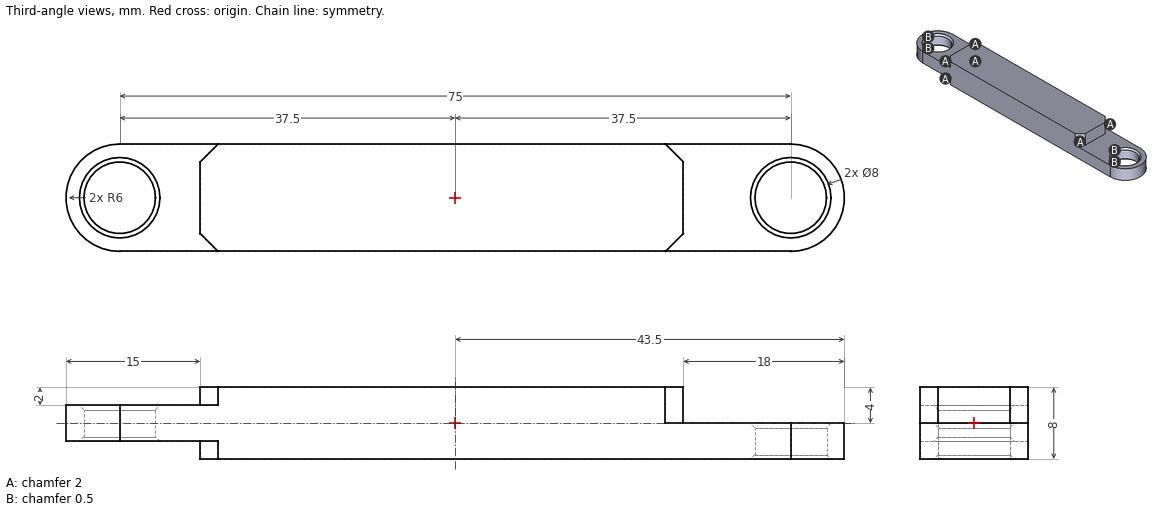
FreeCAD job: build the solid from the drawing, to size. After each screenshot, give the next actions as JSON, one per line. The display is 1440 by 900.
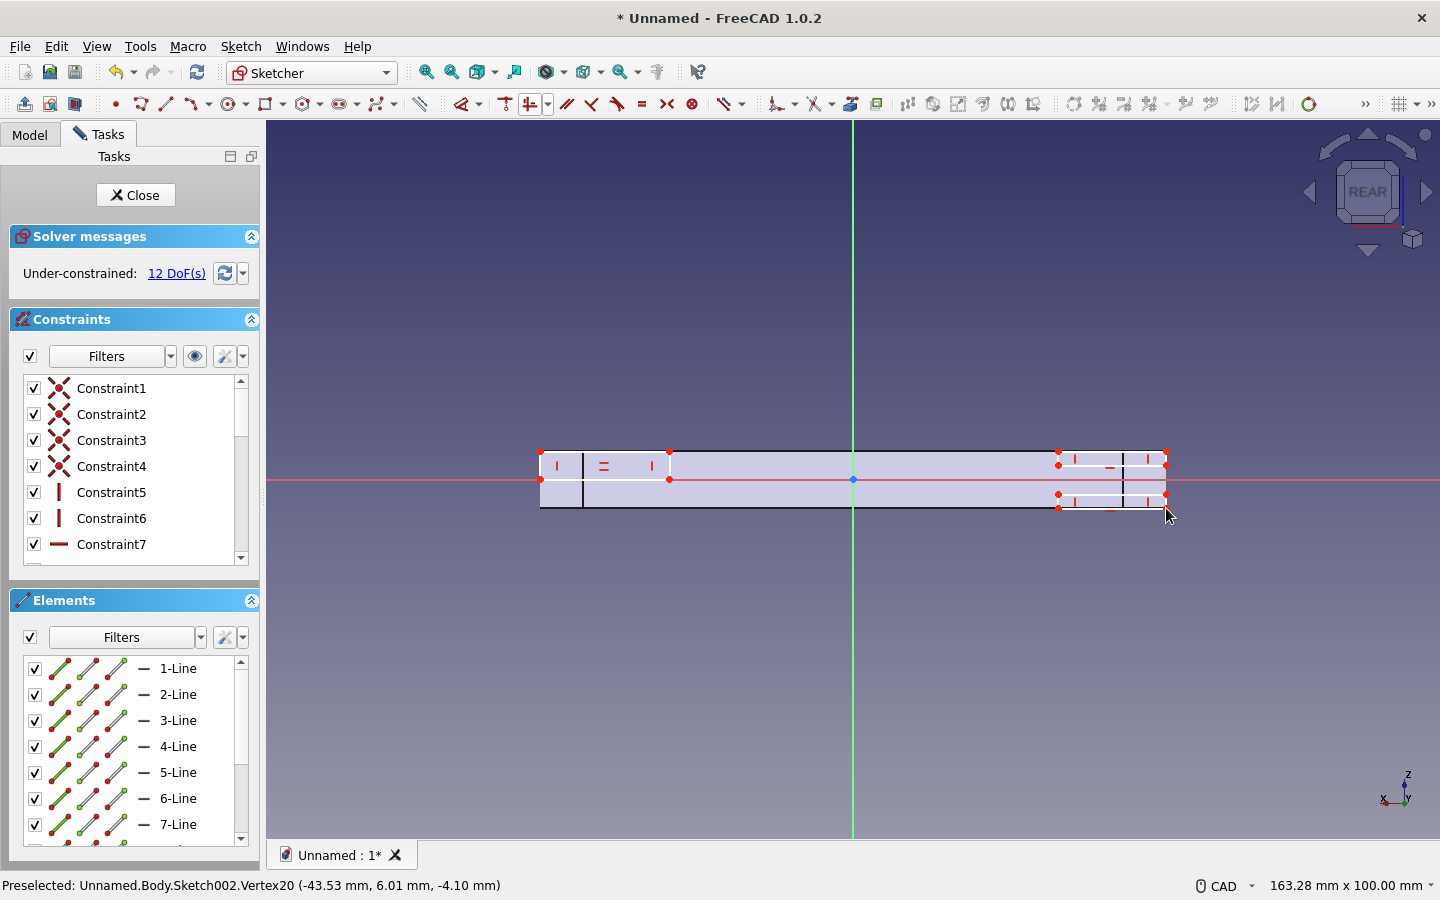
{"action": "left_click", "coordinate": [540, 452]}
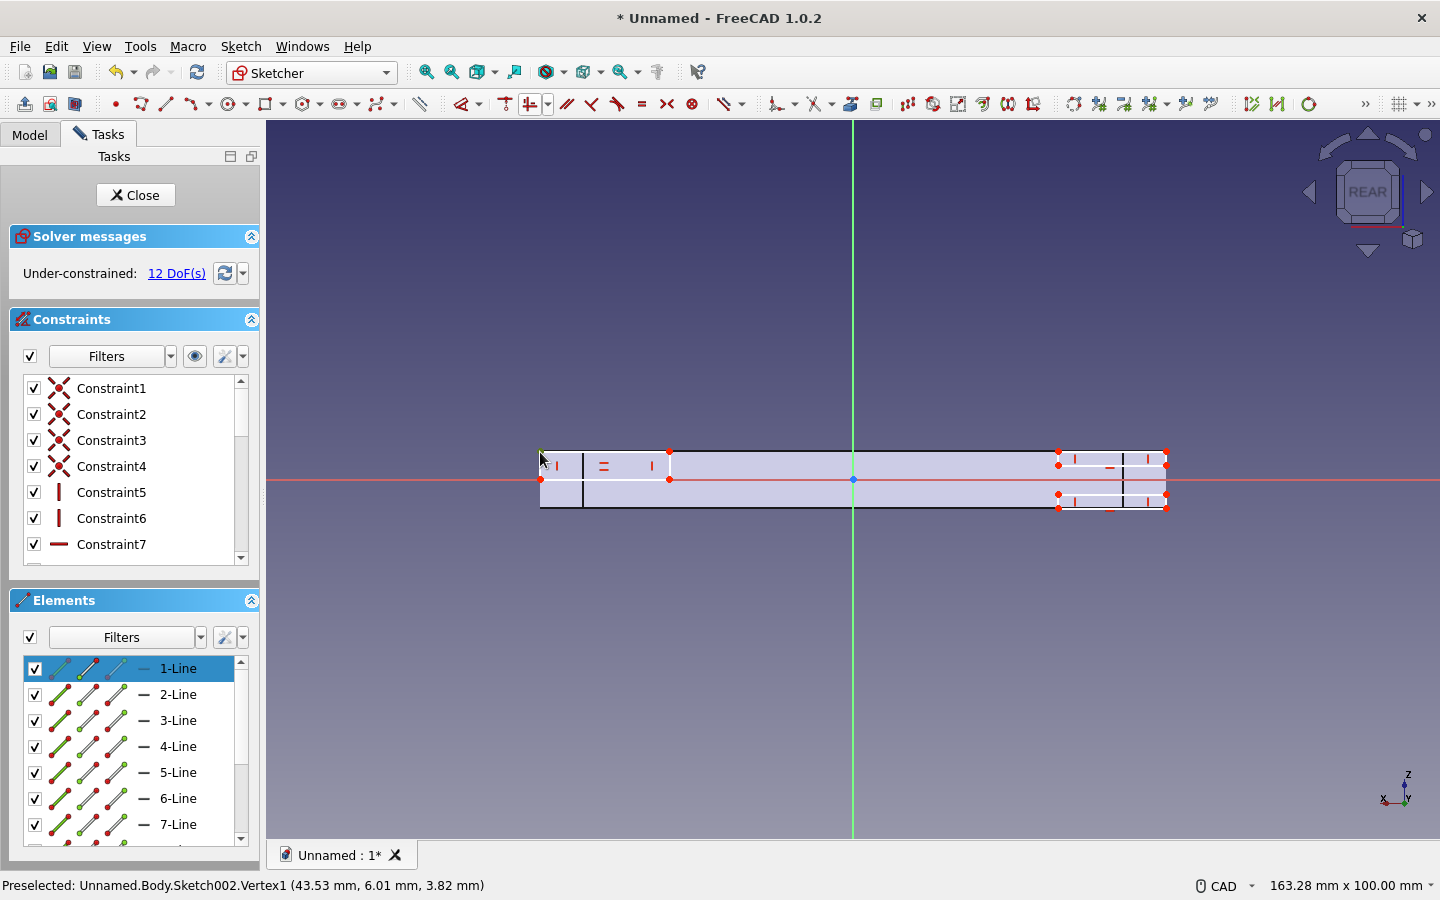
{"action": "left_click", "coordinate": [1166, 452]}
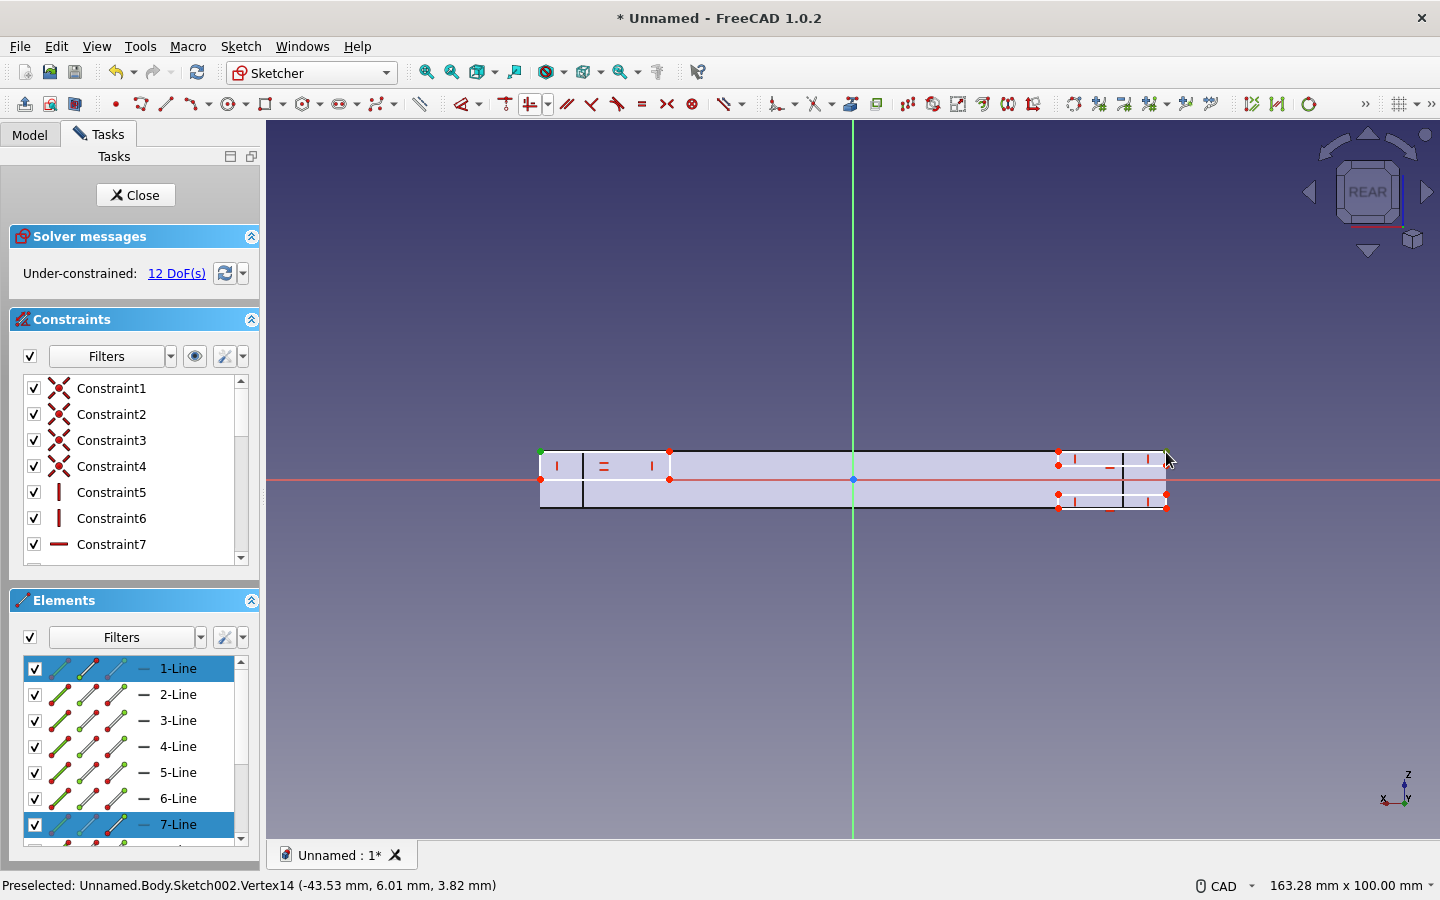
{"action": "left_click", "coordinate": [853, 764]}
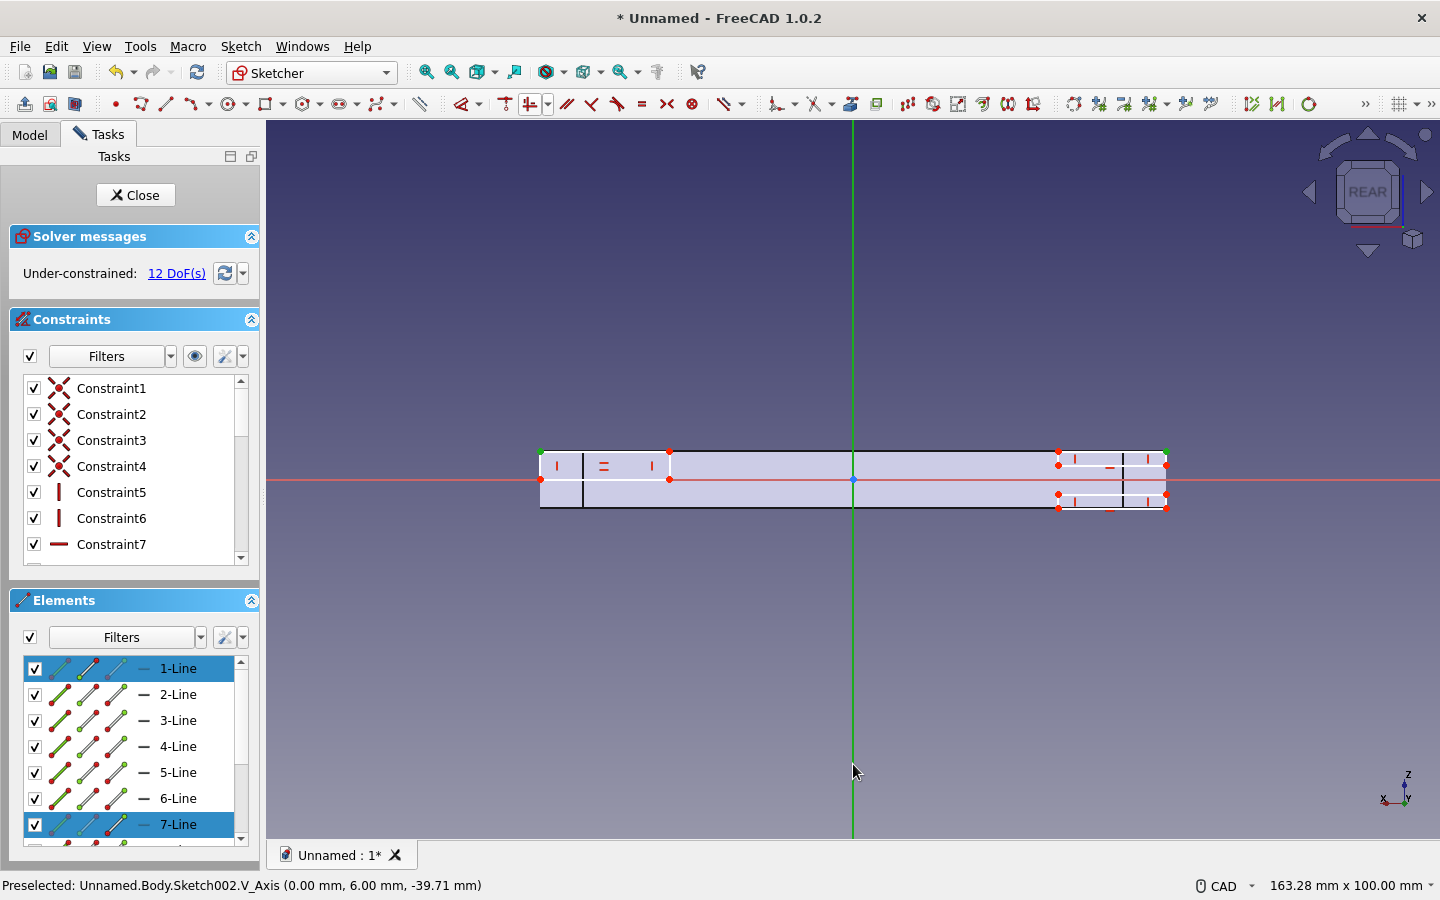
{"action": "left_click", "coordinate": [667, 104]}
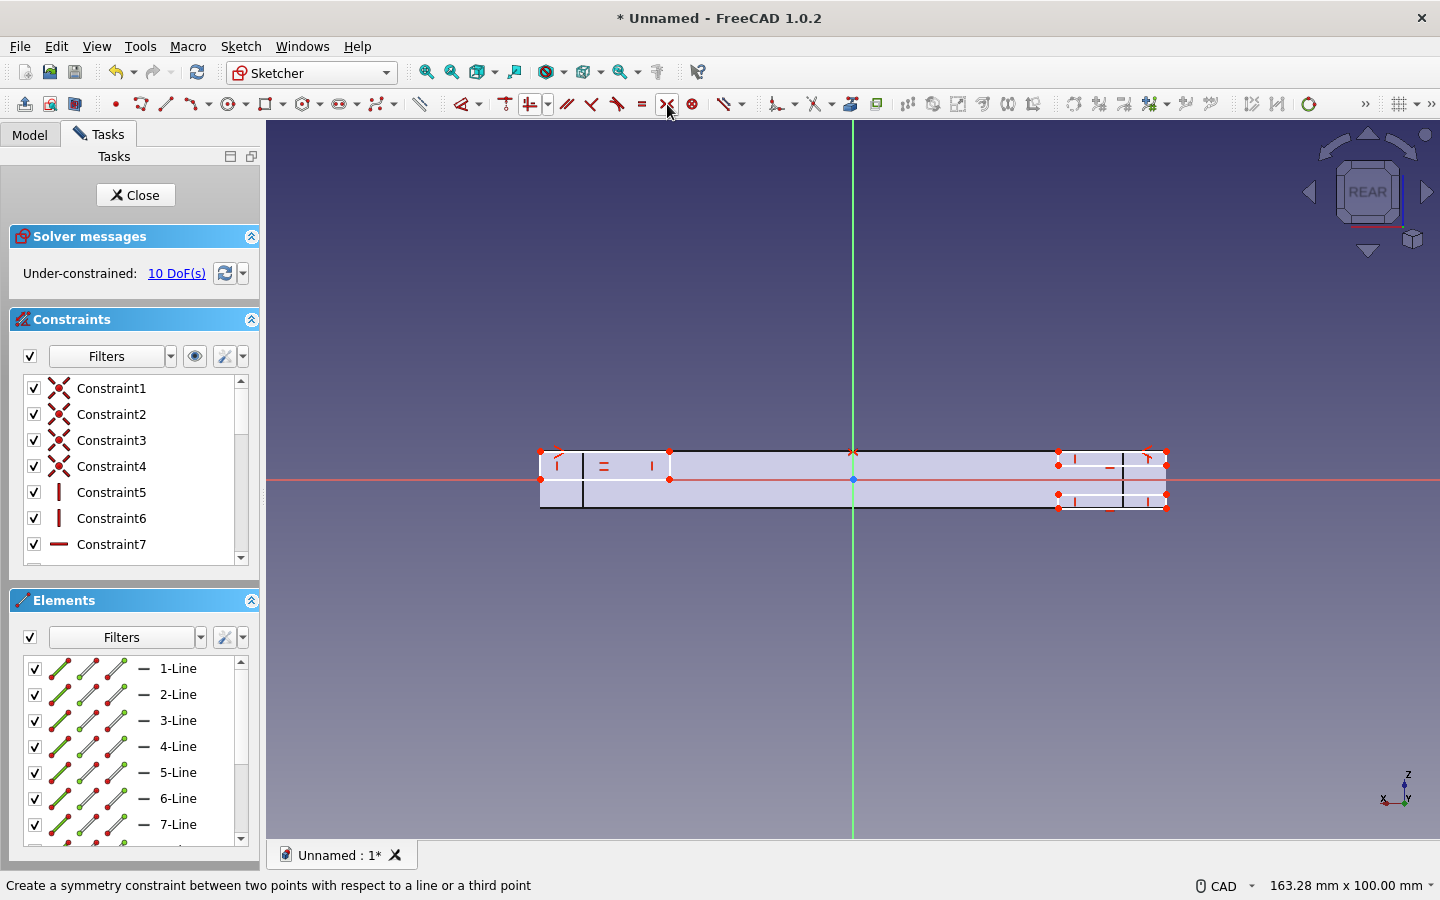
{"action": "left_click", "coordinate": [1058, 466]}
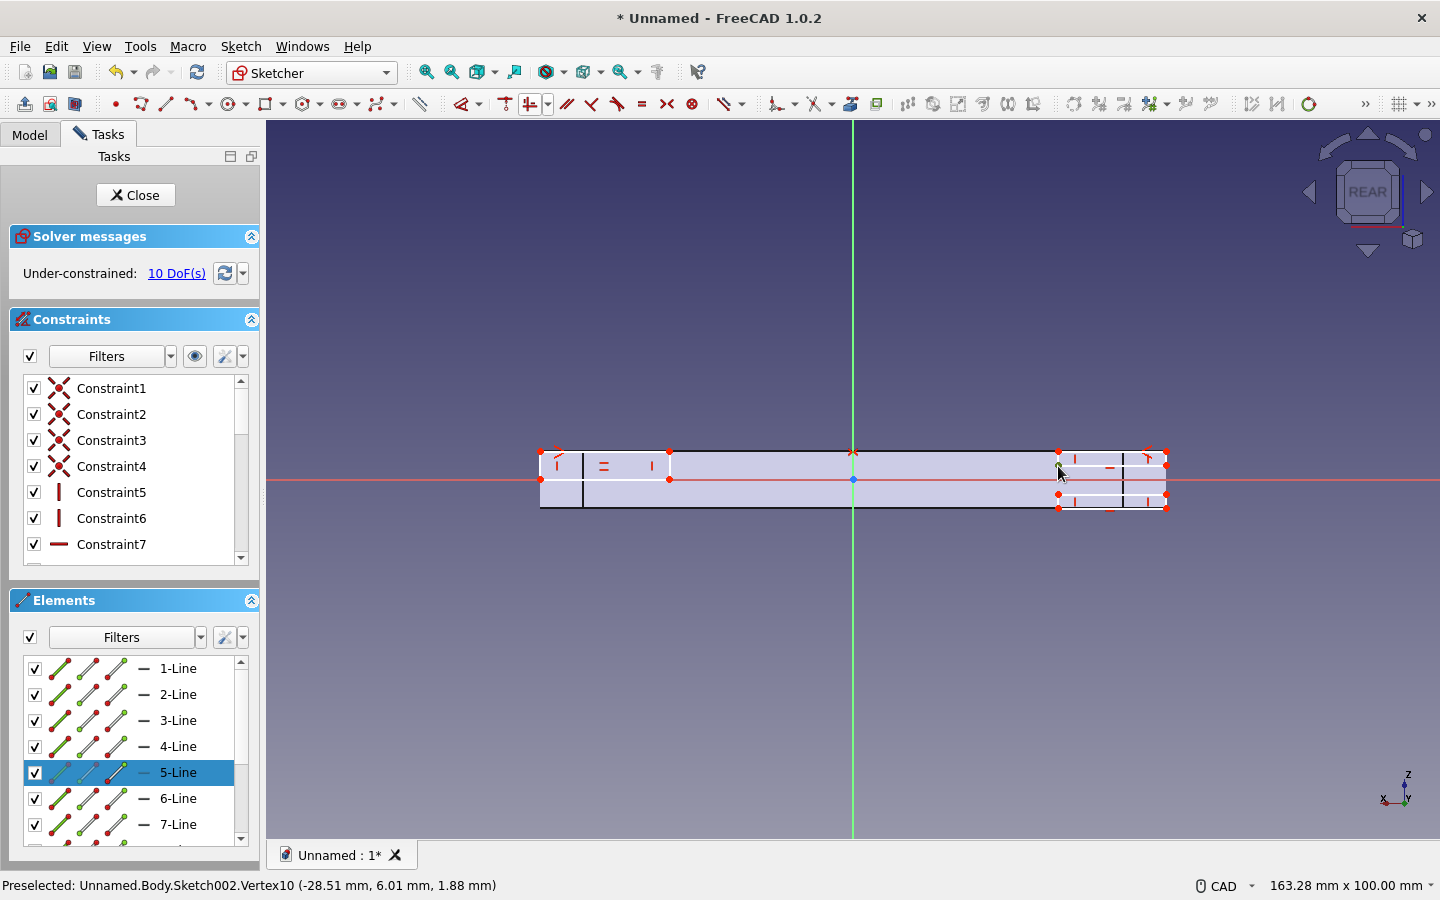
{"action": "left_click", "coordinate": [1058, 495]}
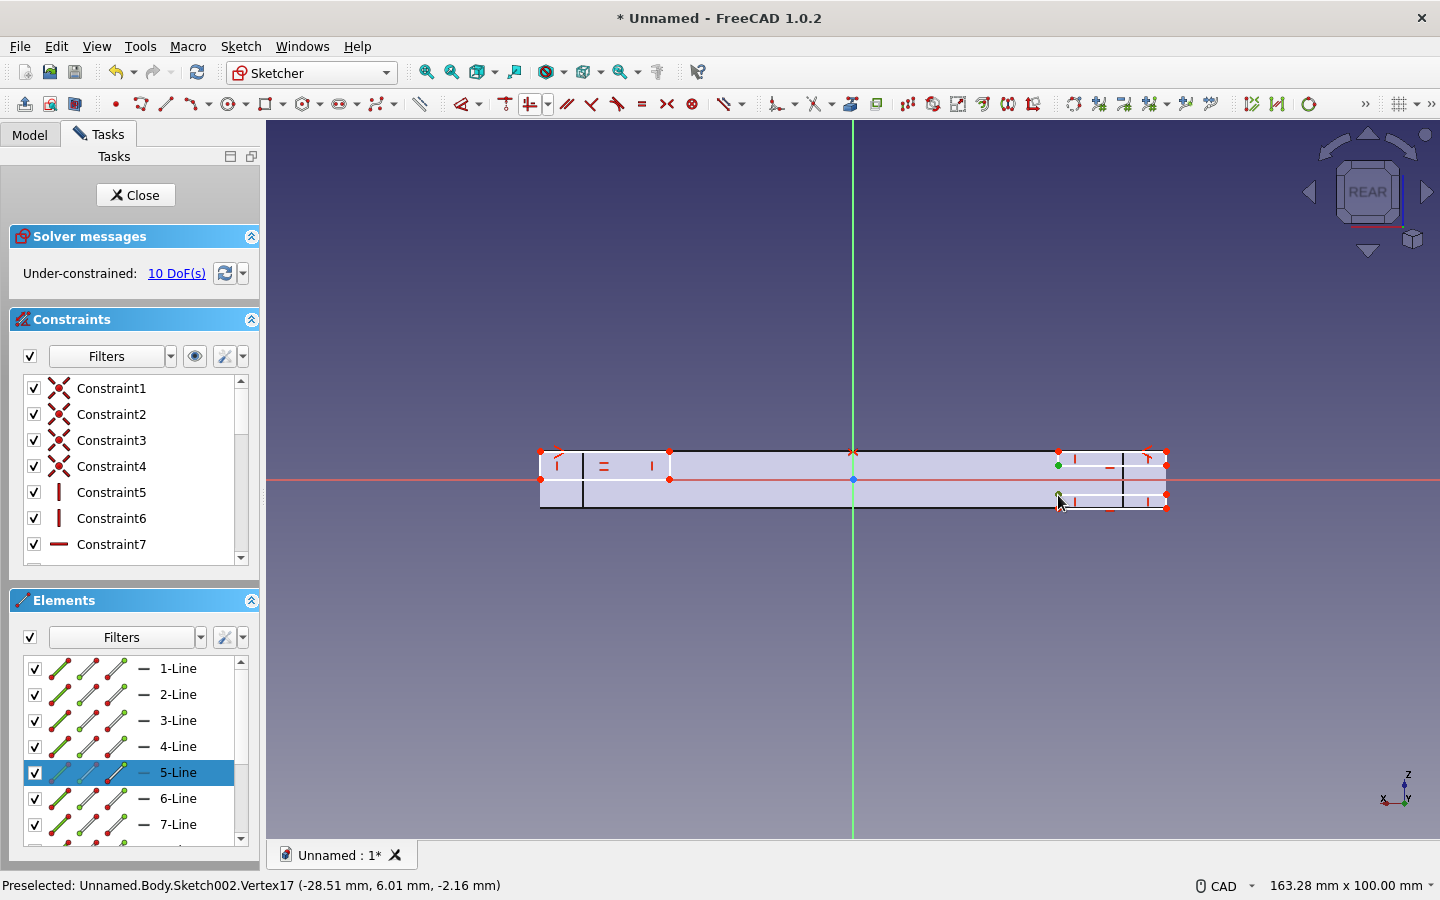
{"action": "left_click", "coordinate": [364, 479]}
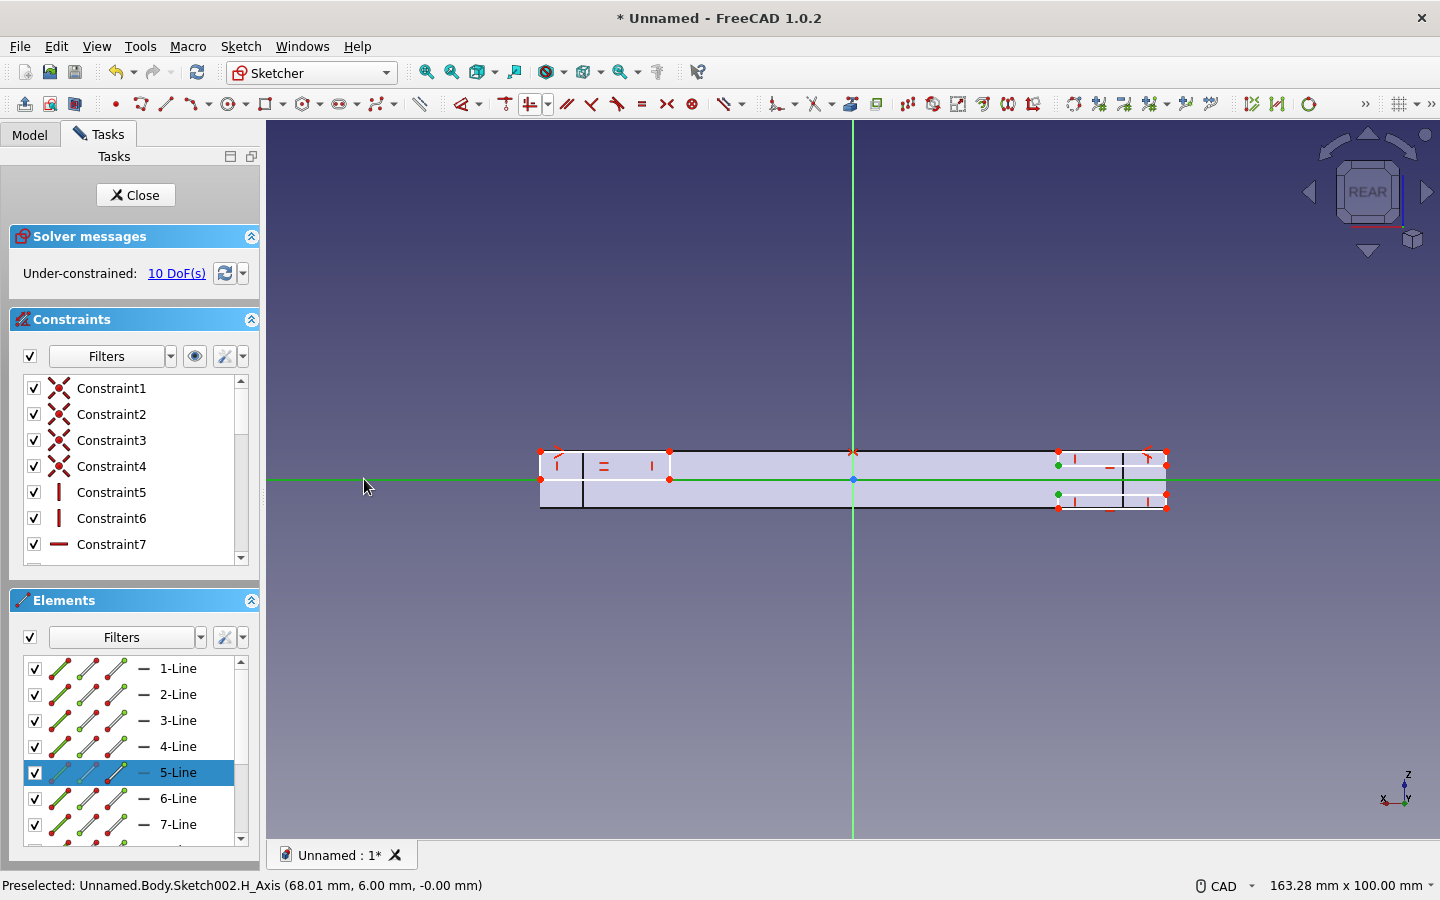
{"action": "left_click", "coordinate": [667, 104]}